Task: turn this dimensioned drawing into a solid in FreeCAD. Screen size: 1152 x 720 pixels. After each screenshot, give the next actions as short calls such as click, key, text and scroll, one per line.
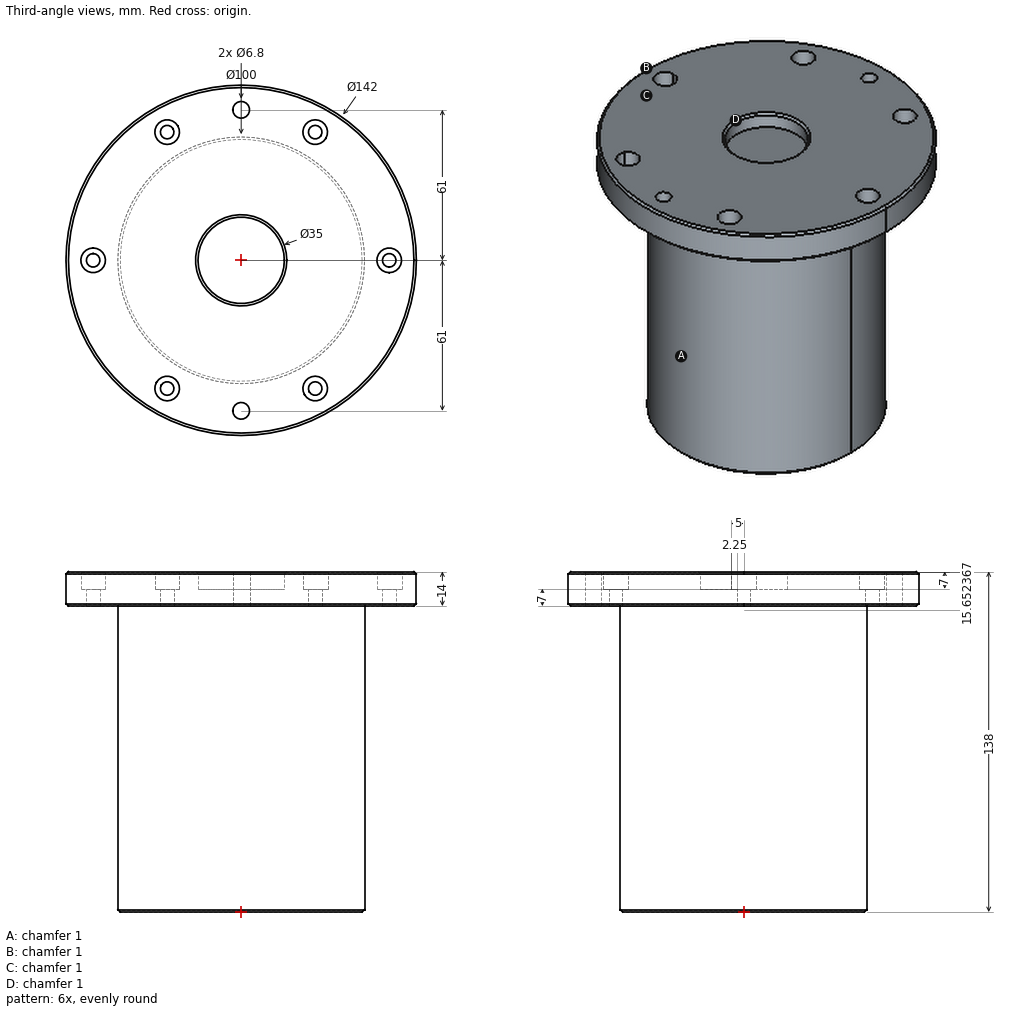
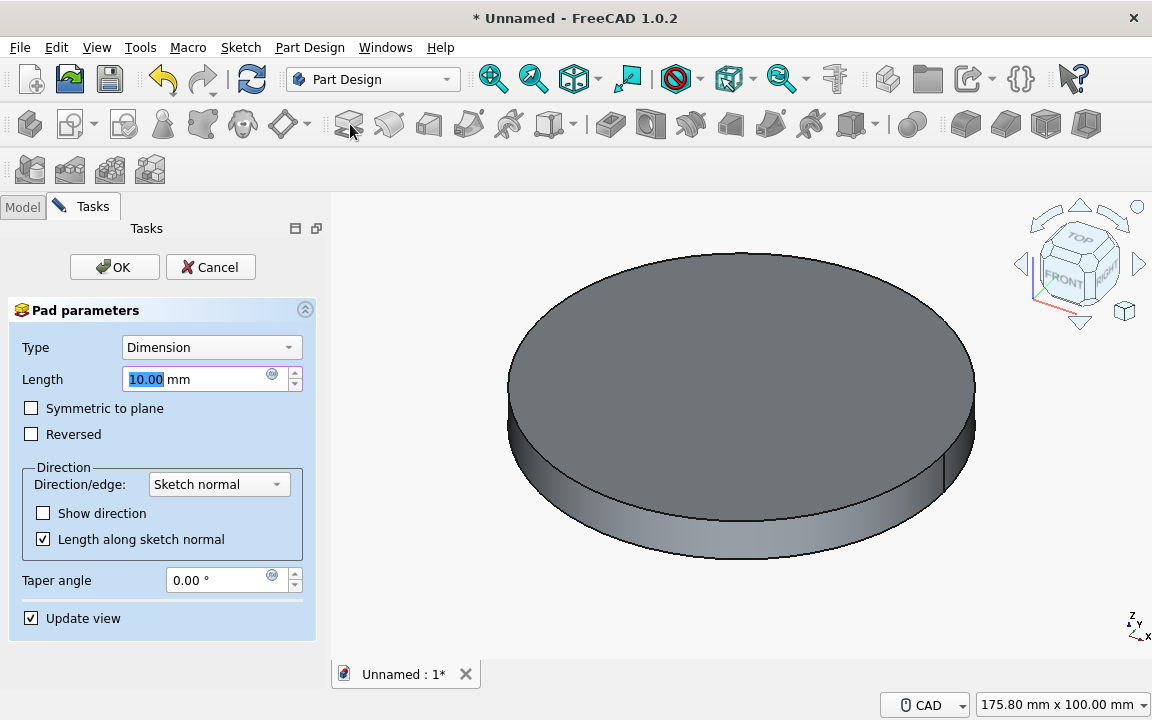
text(138)
key(Tab)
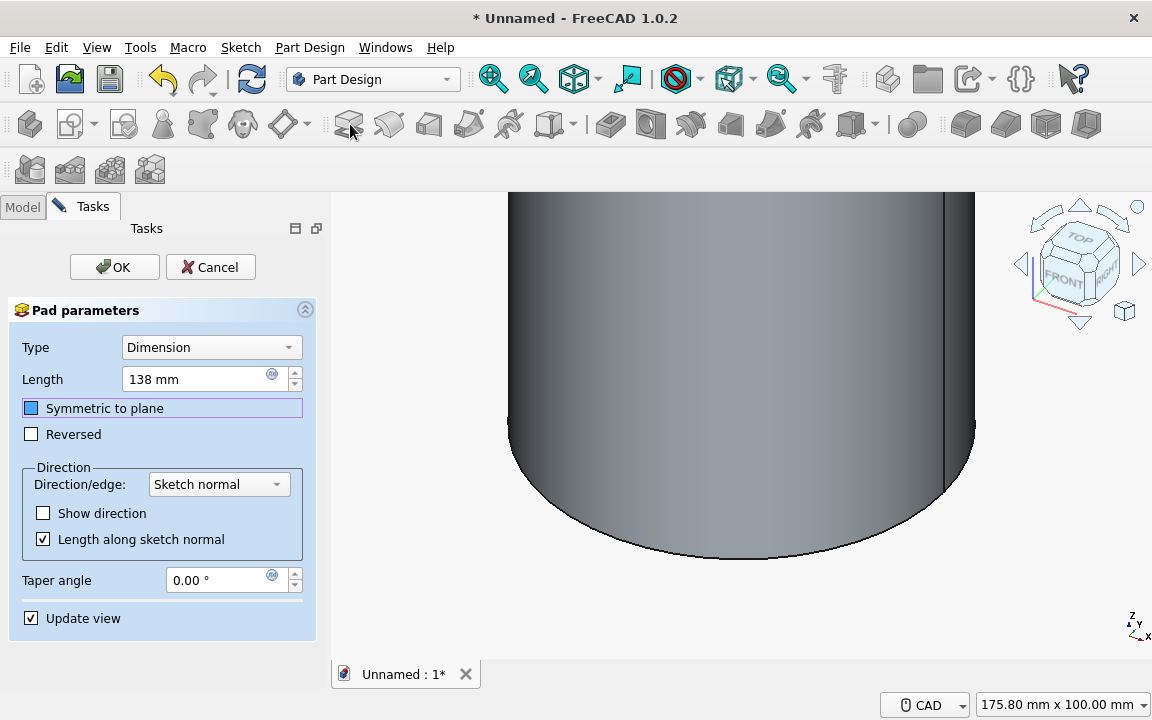
click(115, 267)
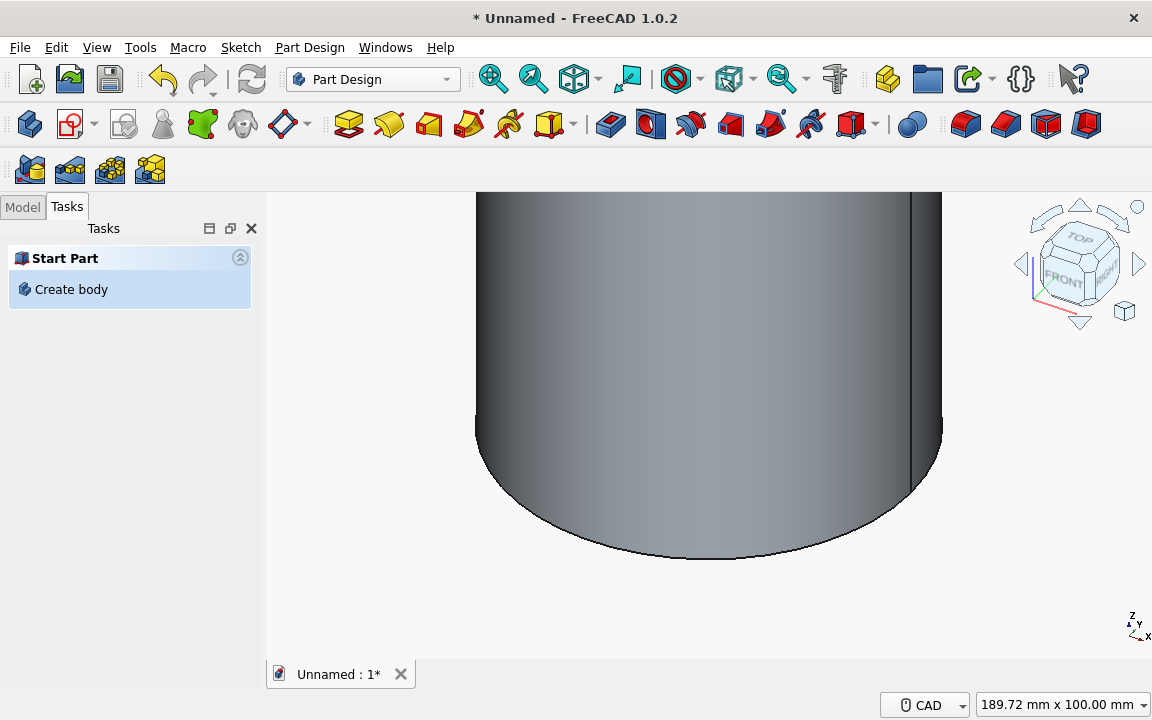
key(v)
key(f)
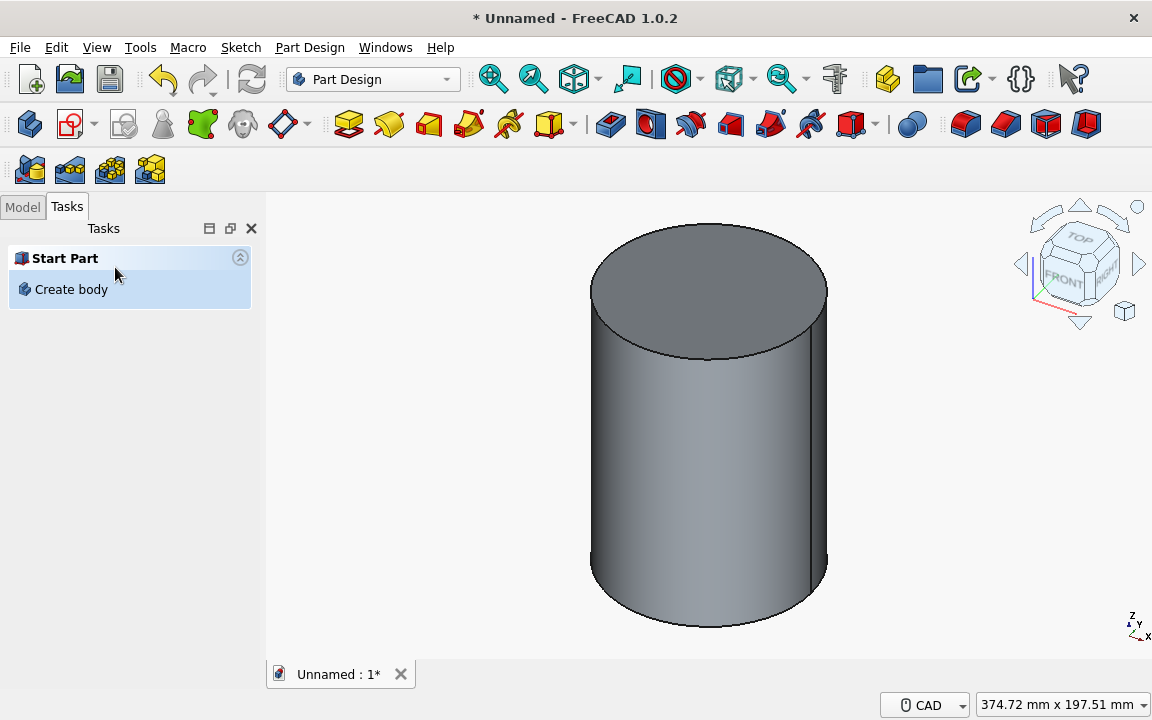
click(23, 206)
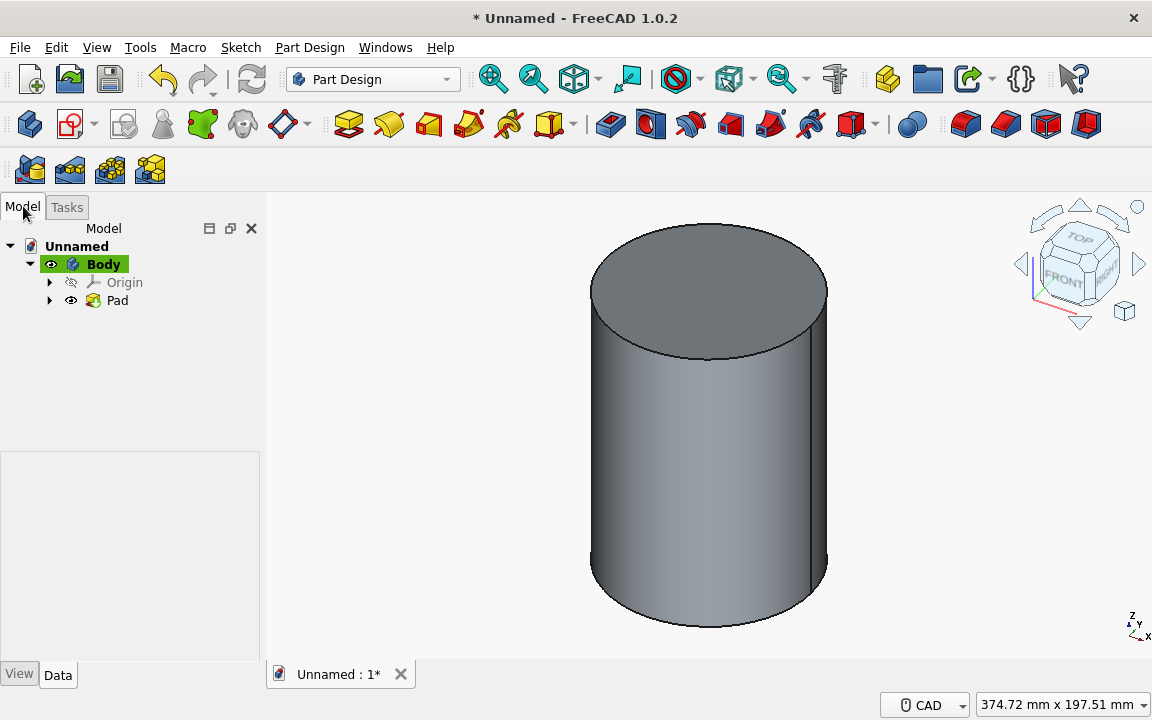
click(50, 282)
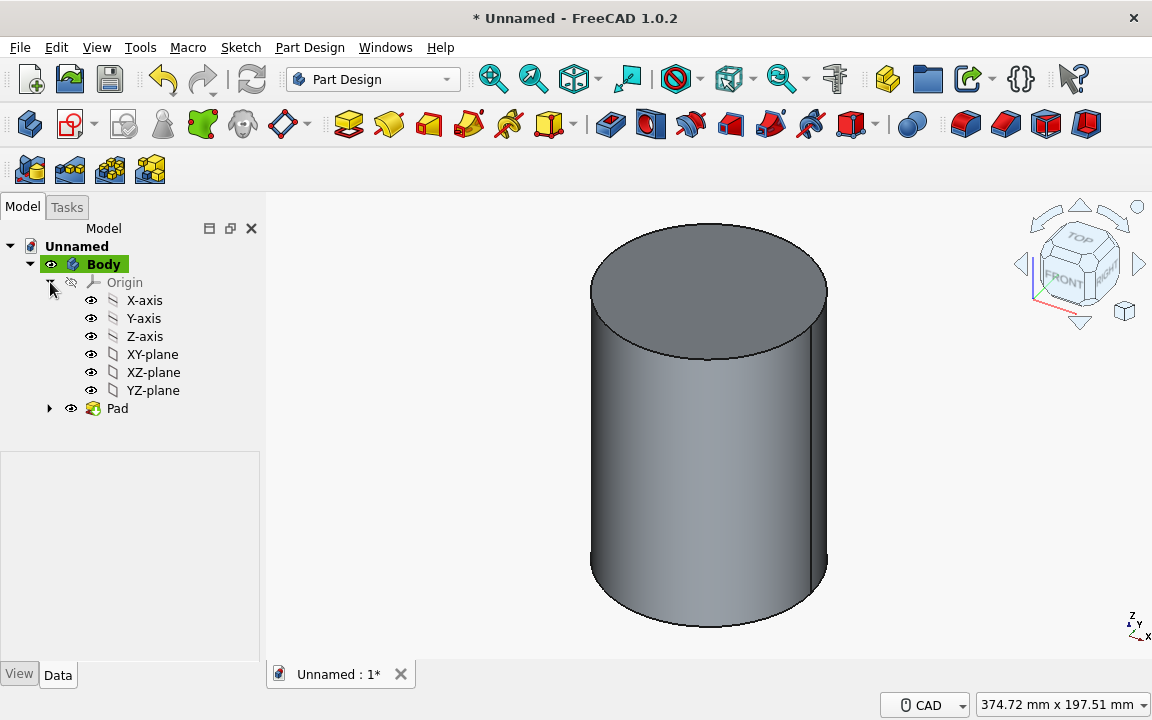
click(136, 354)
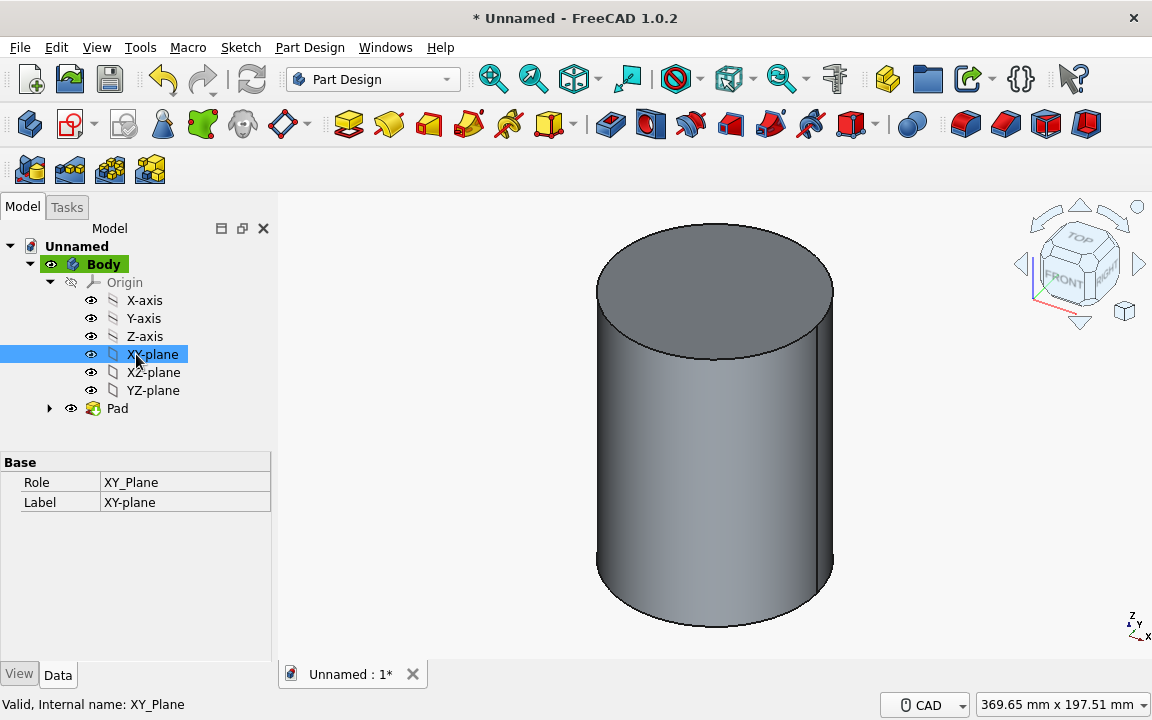
click(284, 124)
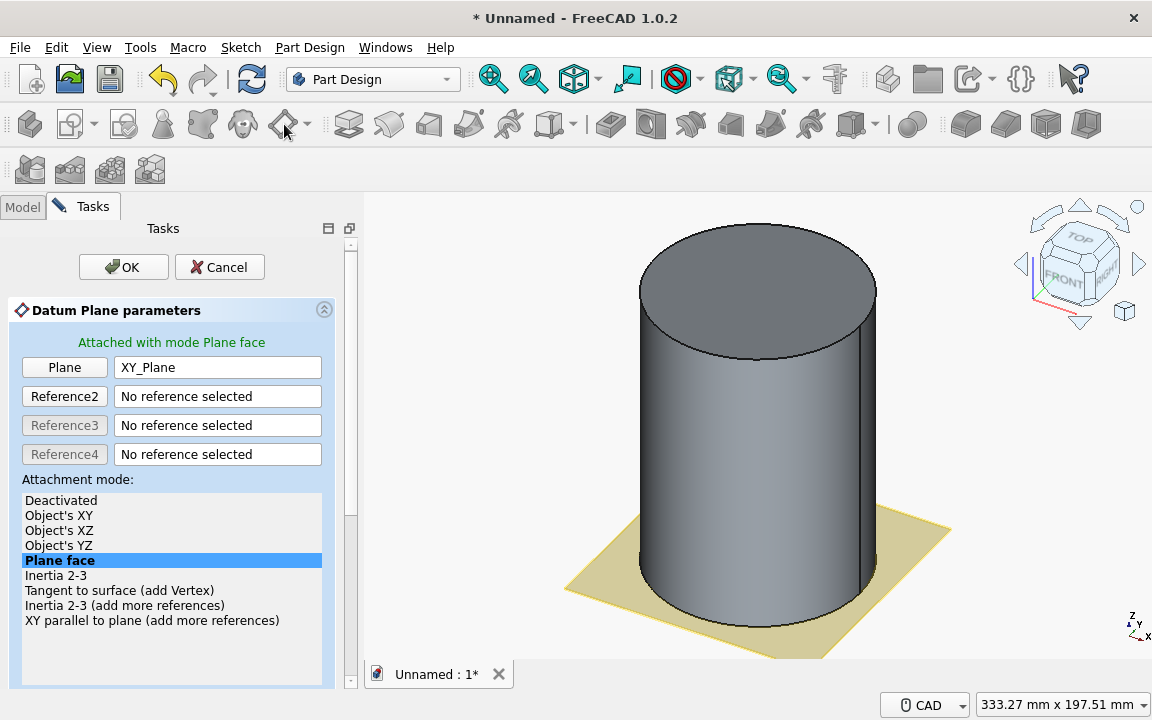
scroll(351, 463, down, 3)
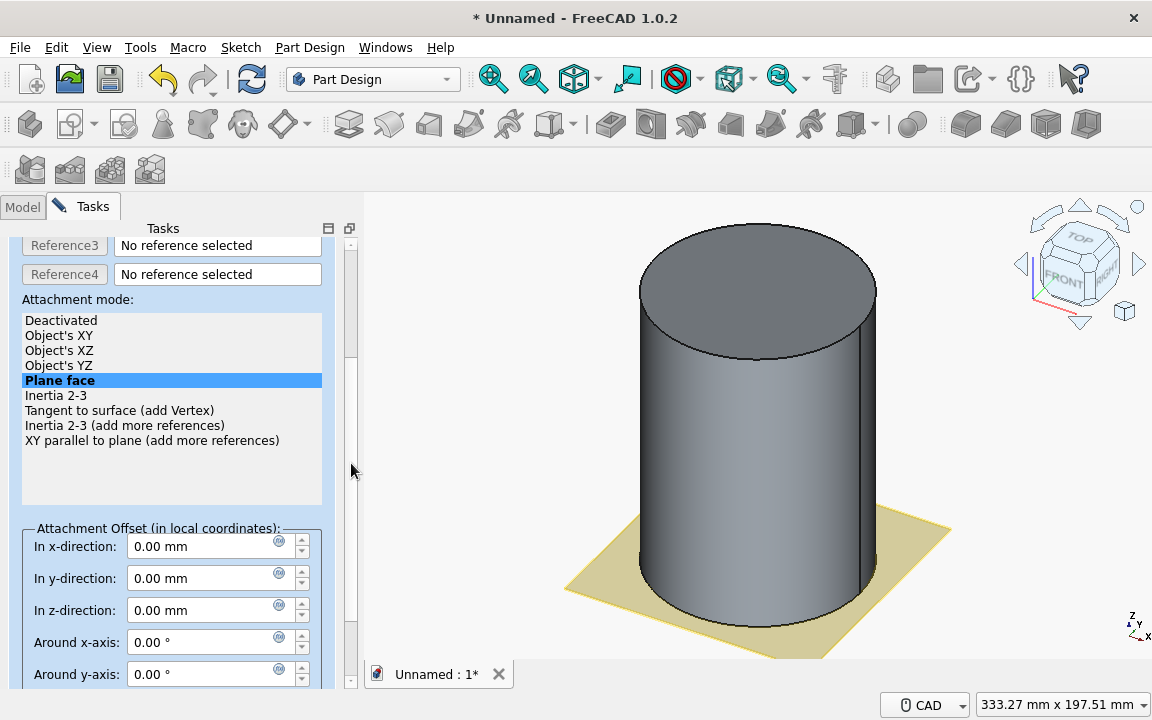
triple_click(210, 610)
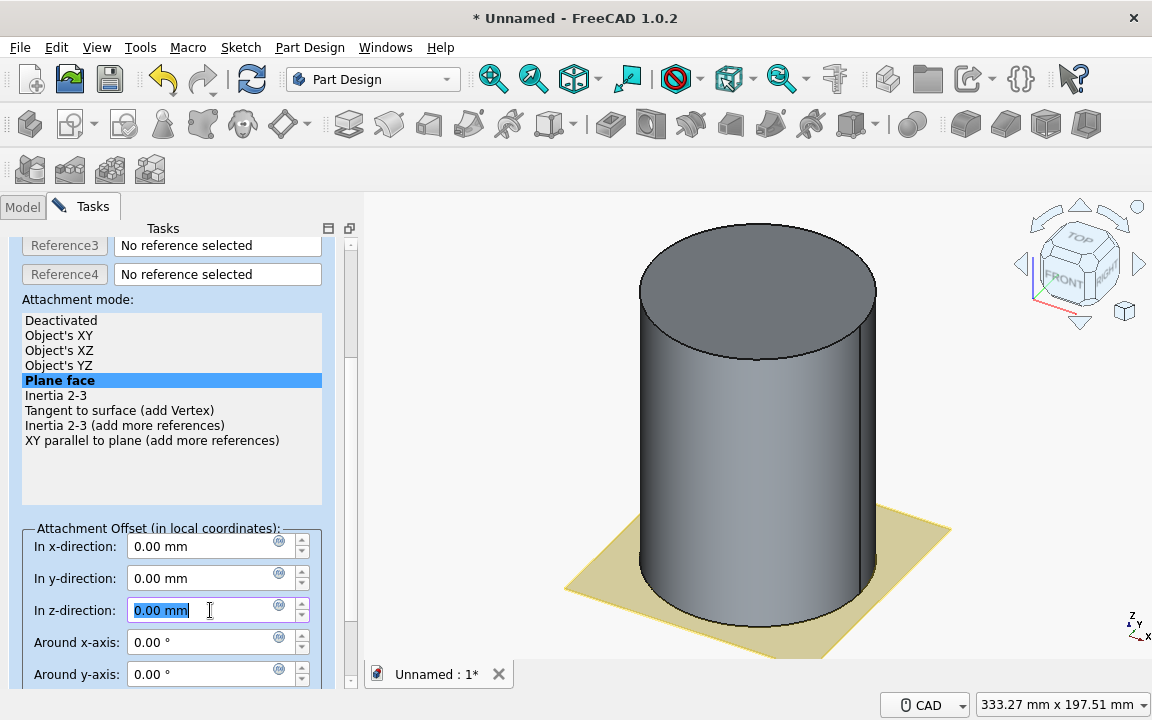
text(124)
key(Tab)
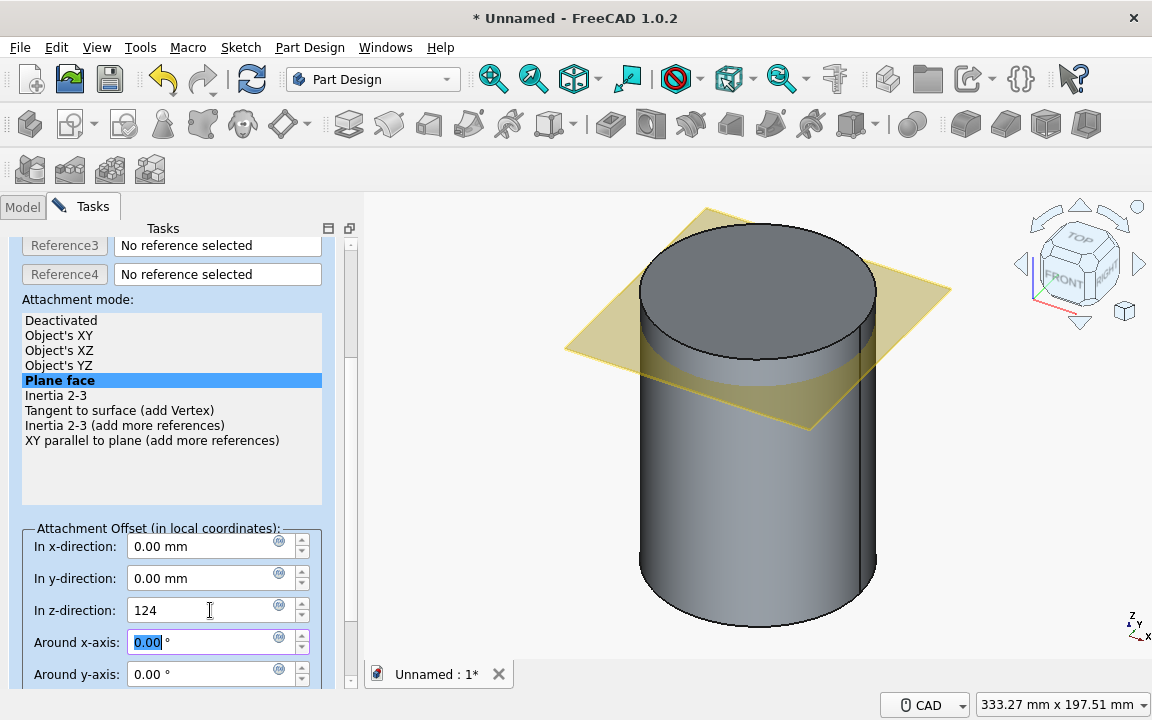
scroll(351, 463, up, 4)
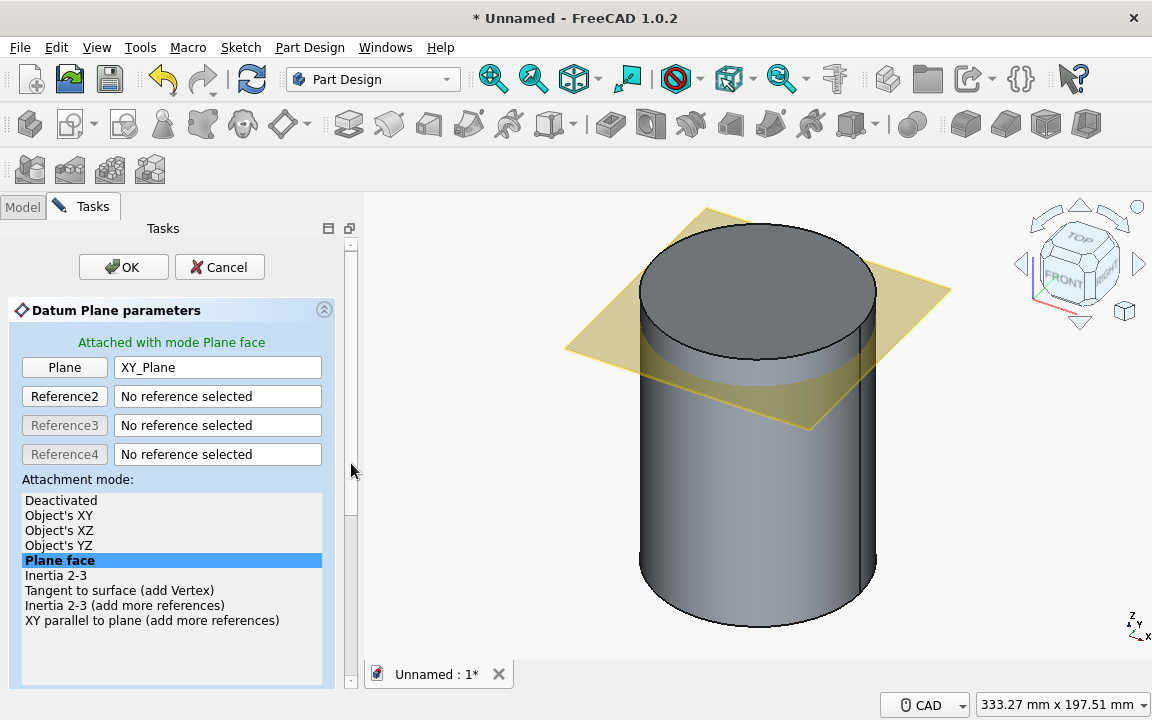
click(124, 267)